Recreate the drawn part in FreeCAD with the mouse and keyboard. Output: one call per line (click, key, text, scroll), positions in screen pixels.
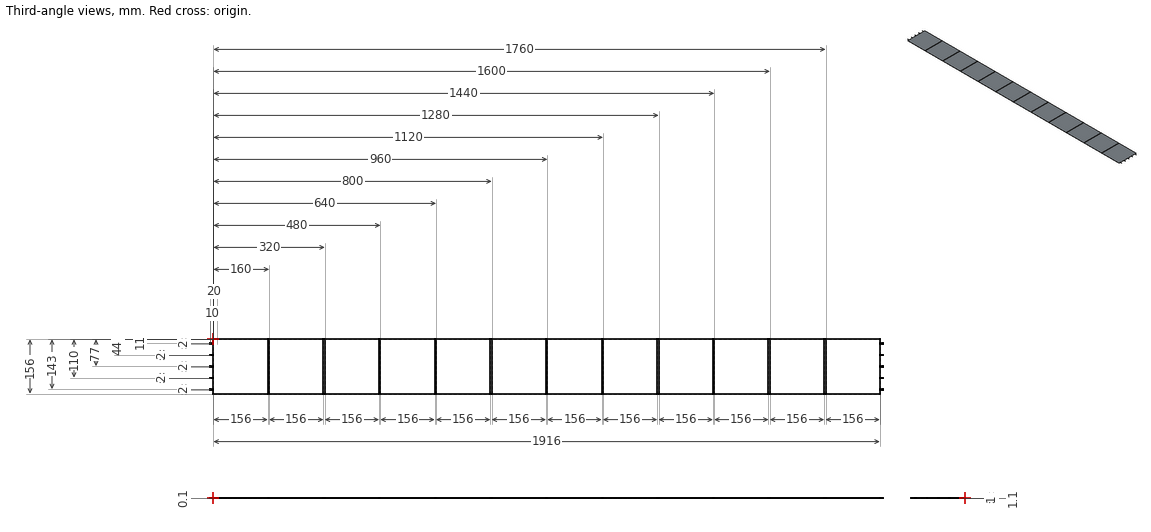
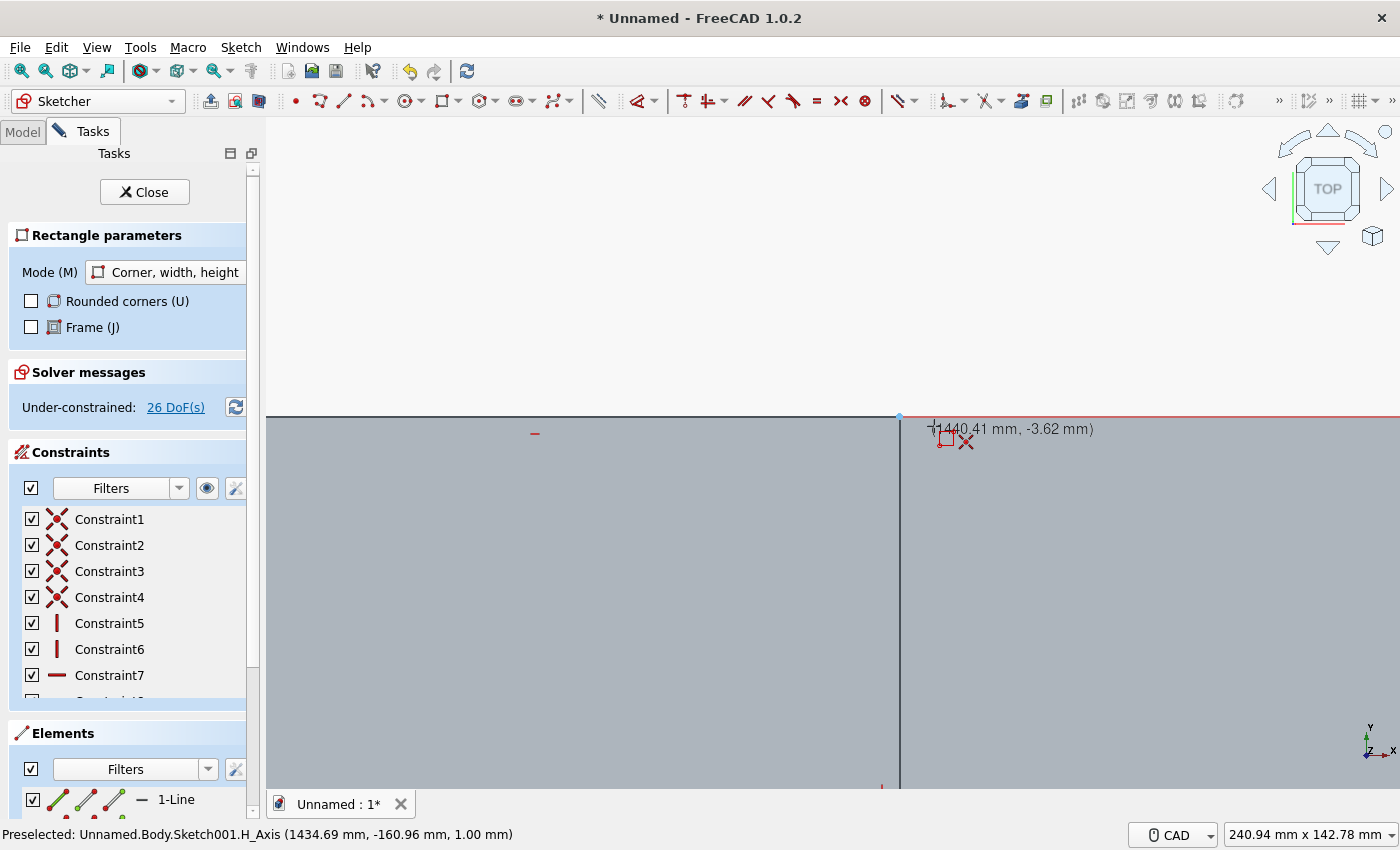
click(925, 417)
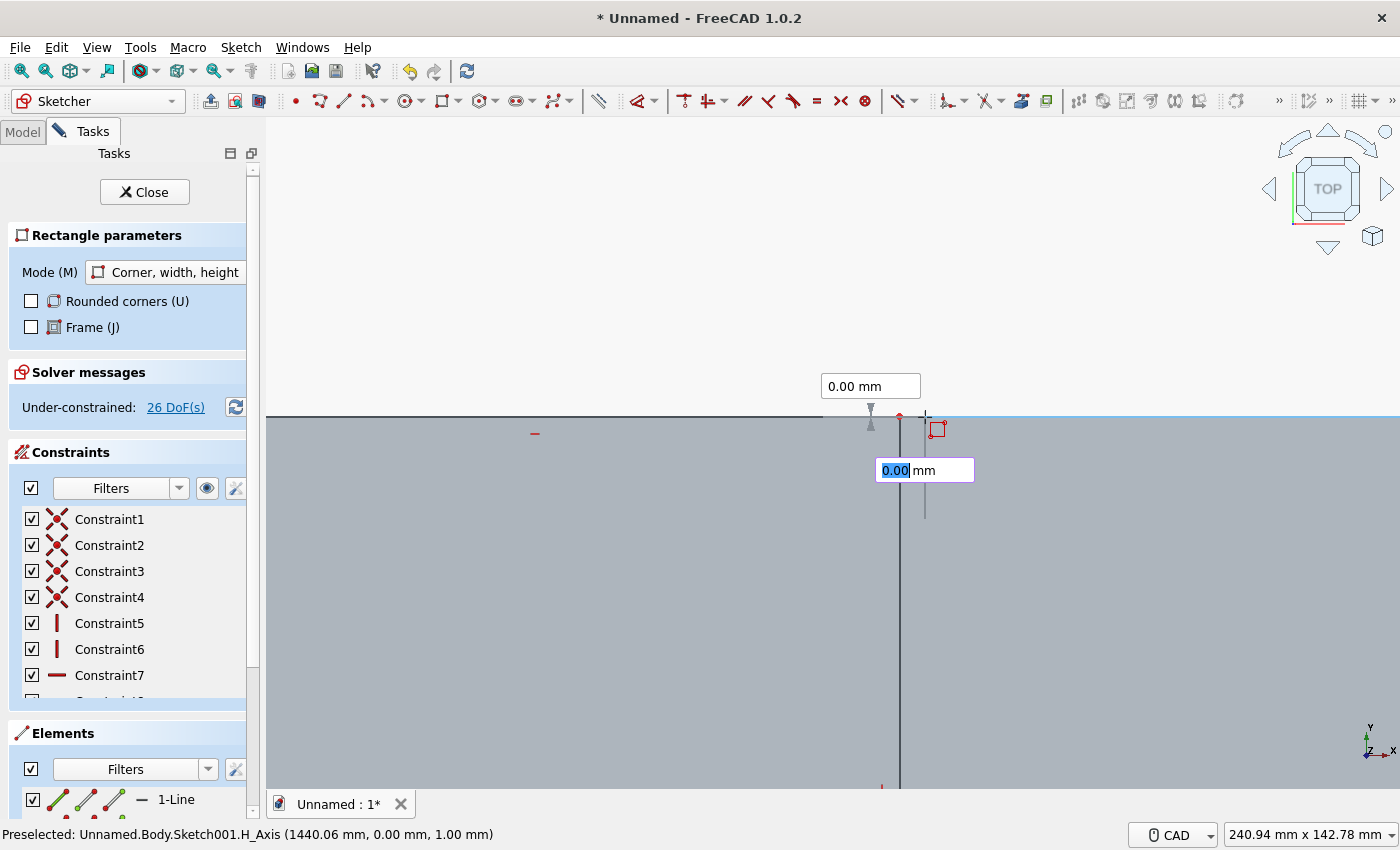
scroll(934, 426, down, 13)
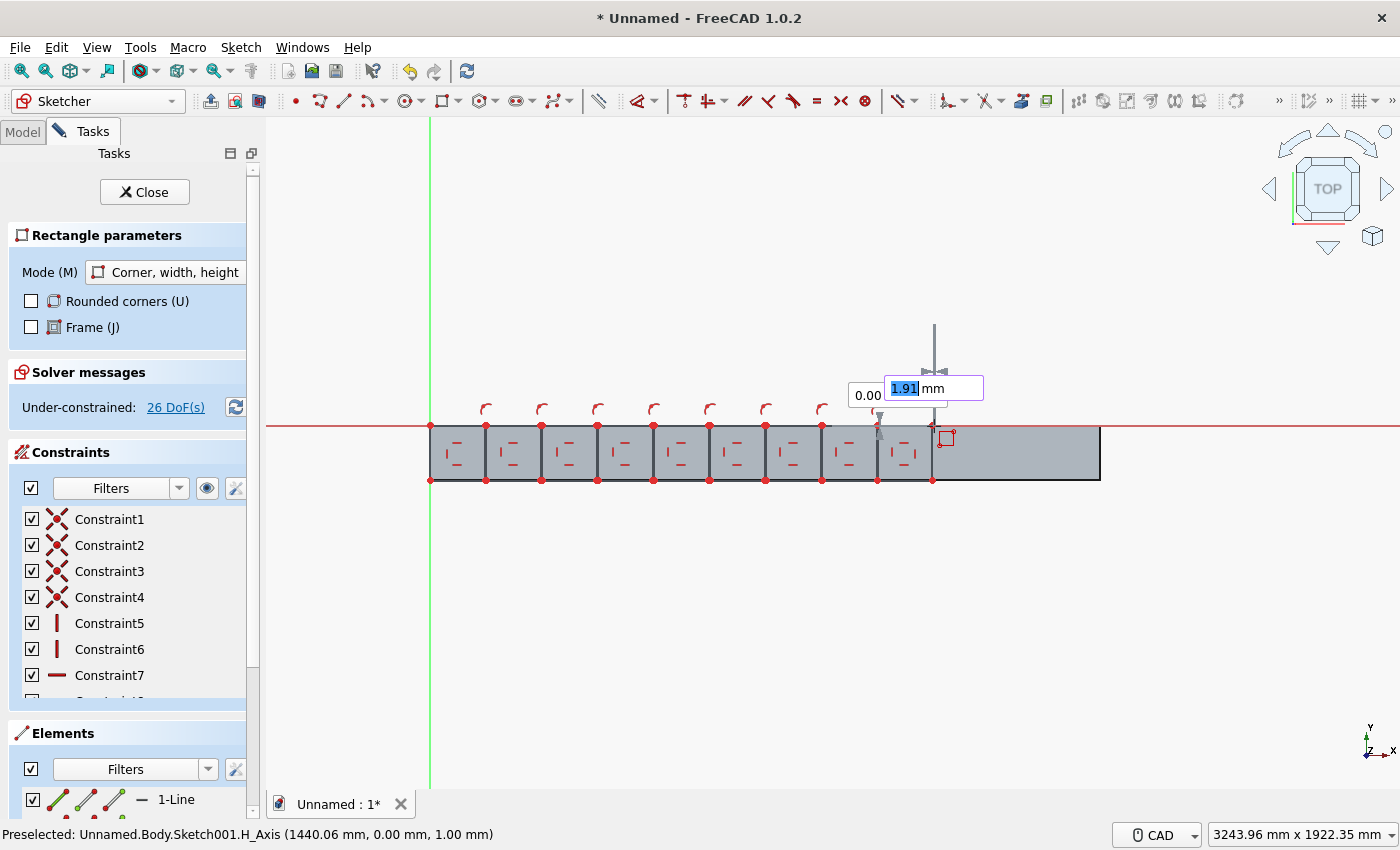
click(988, 480)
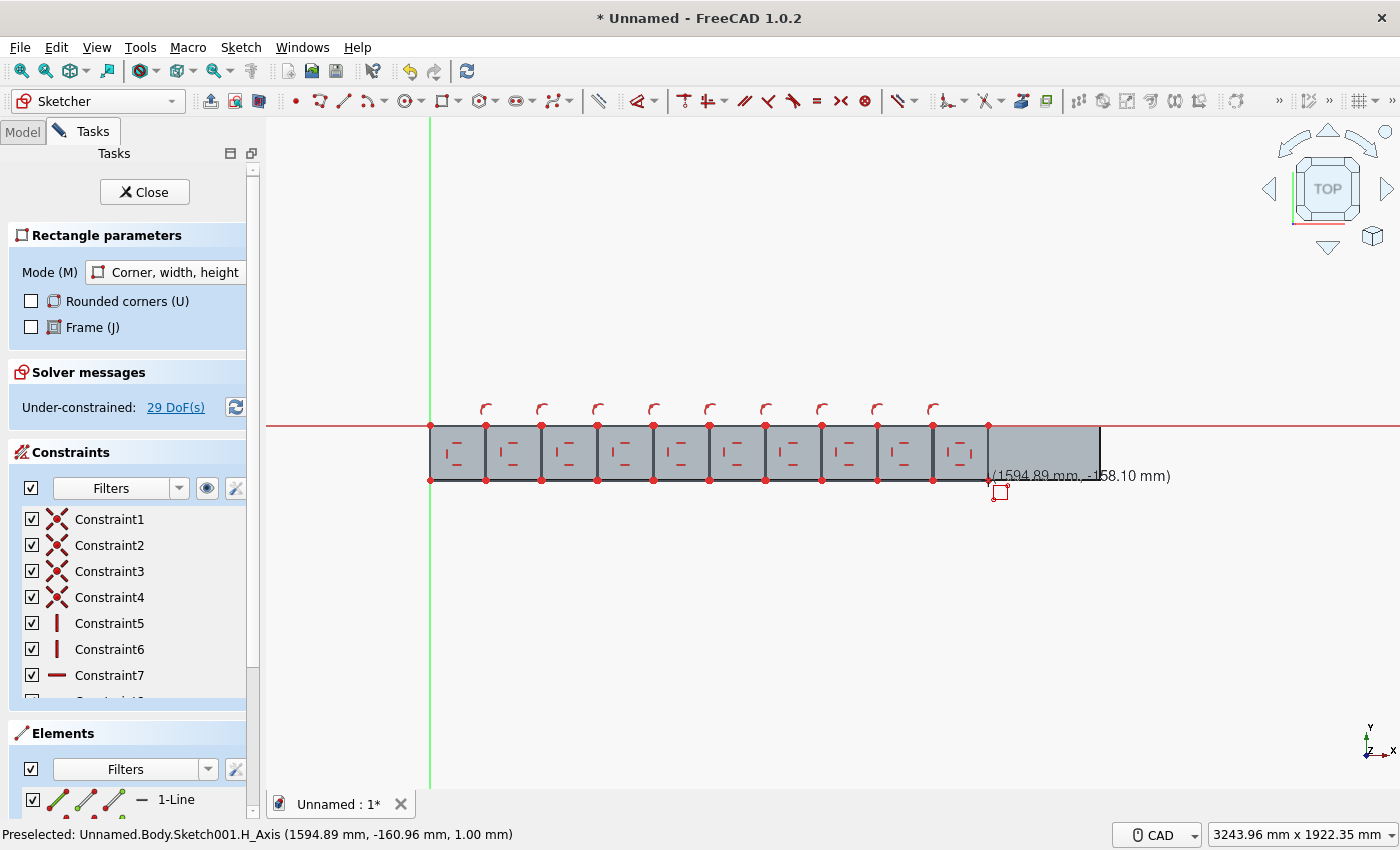
scroll(990, 426, up, 13)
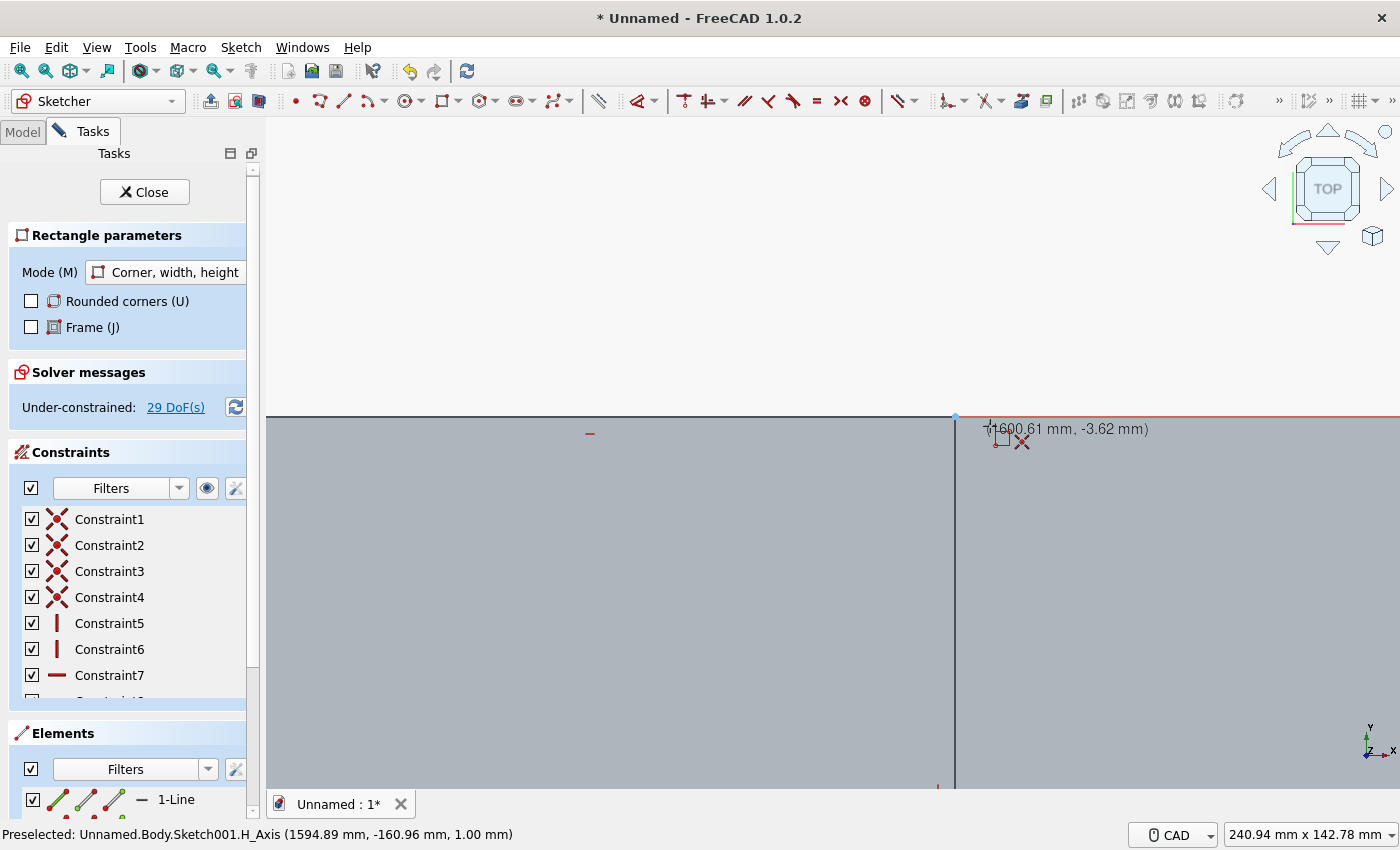
click(979, 417)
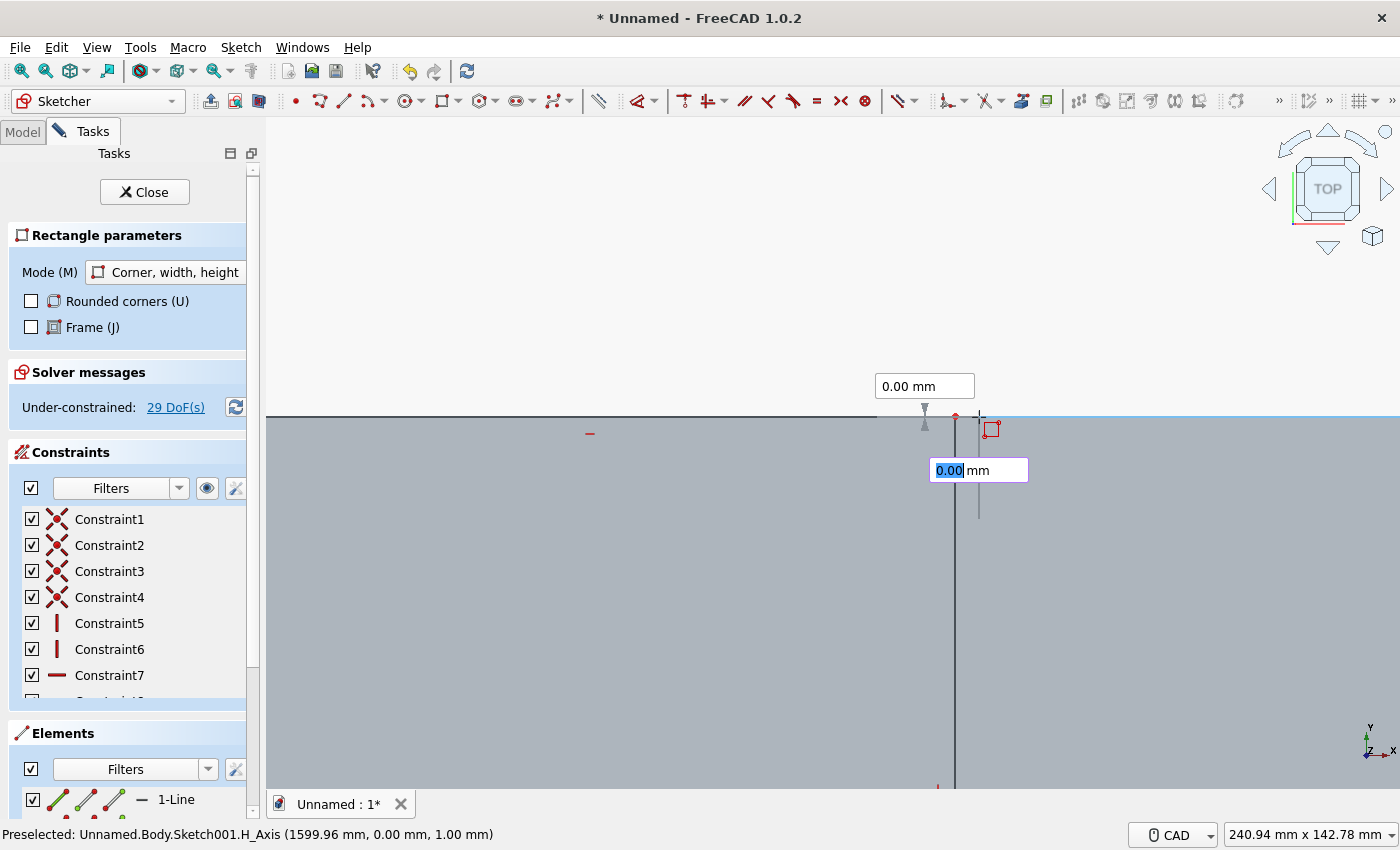
scroll(990, 426, down, 13)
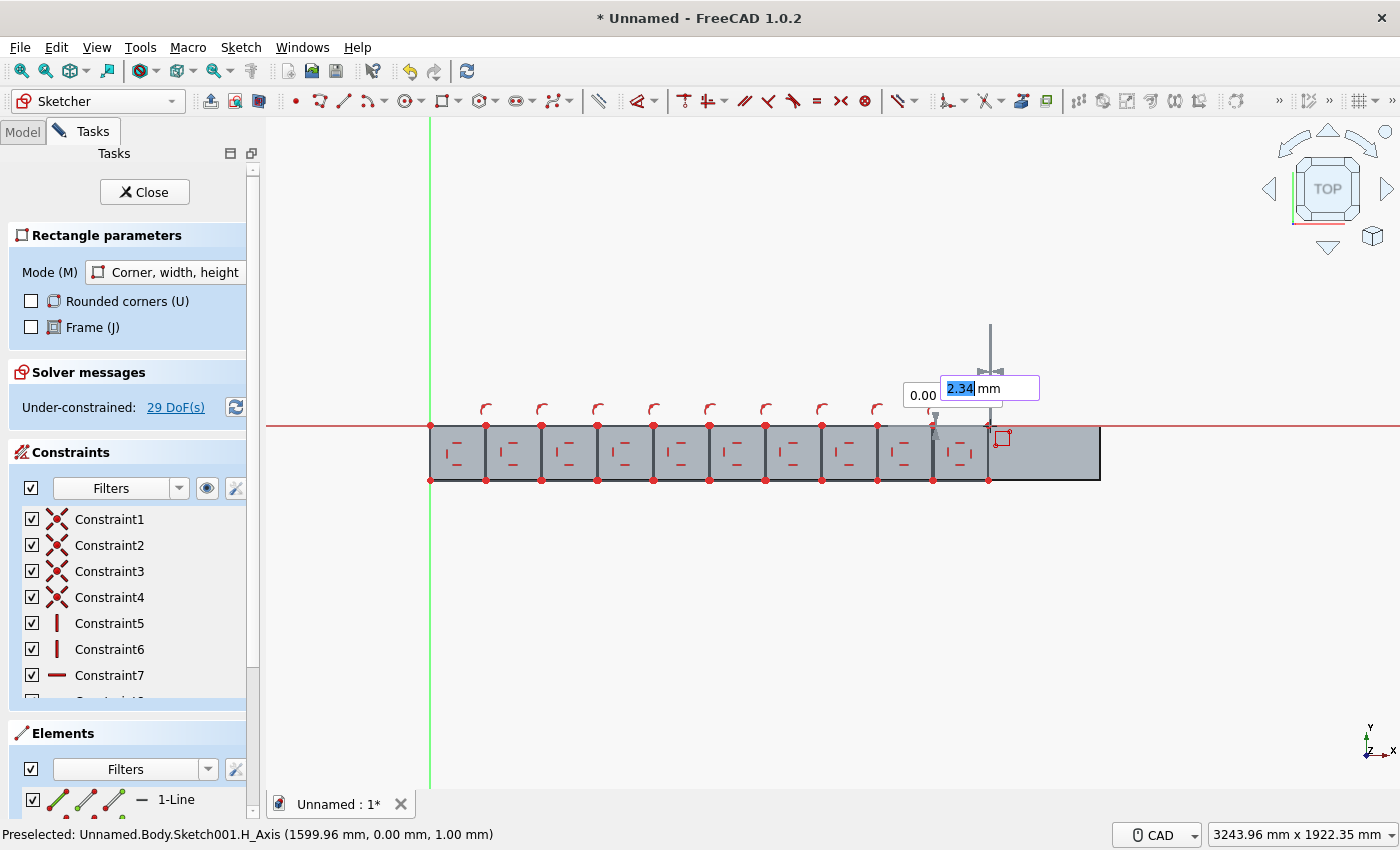
click(1044, 480)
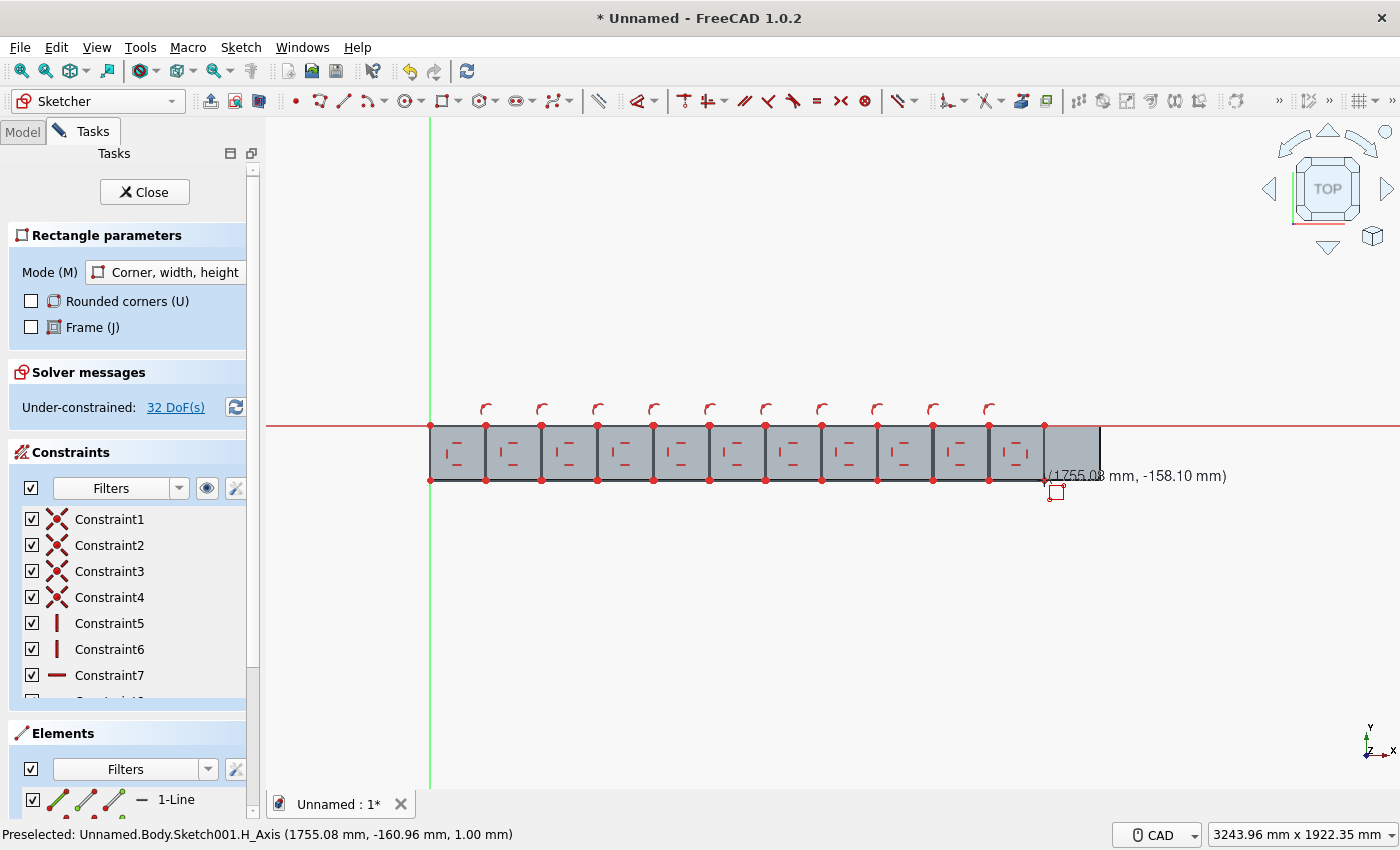
scroll(1046, 426, up, 13)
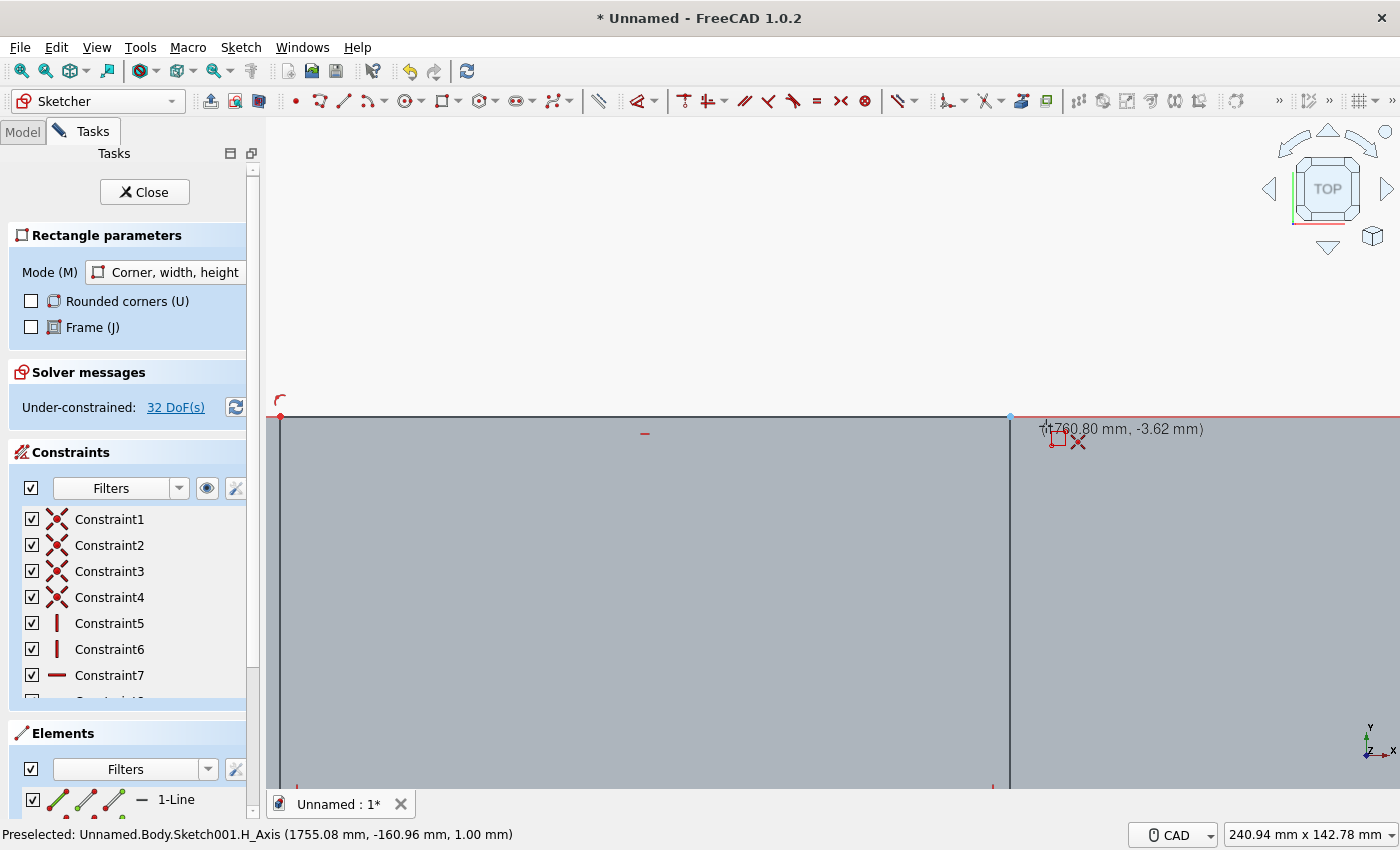
click(1034, 417)